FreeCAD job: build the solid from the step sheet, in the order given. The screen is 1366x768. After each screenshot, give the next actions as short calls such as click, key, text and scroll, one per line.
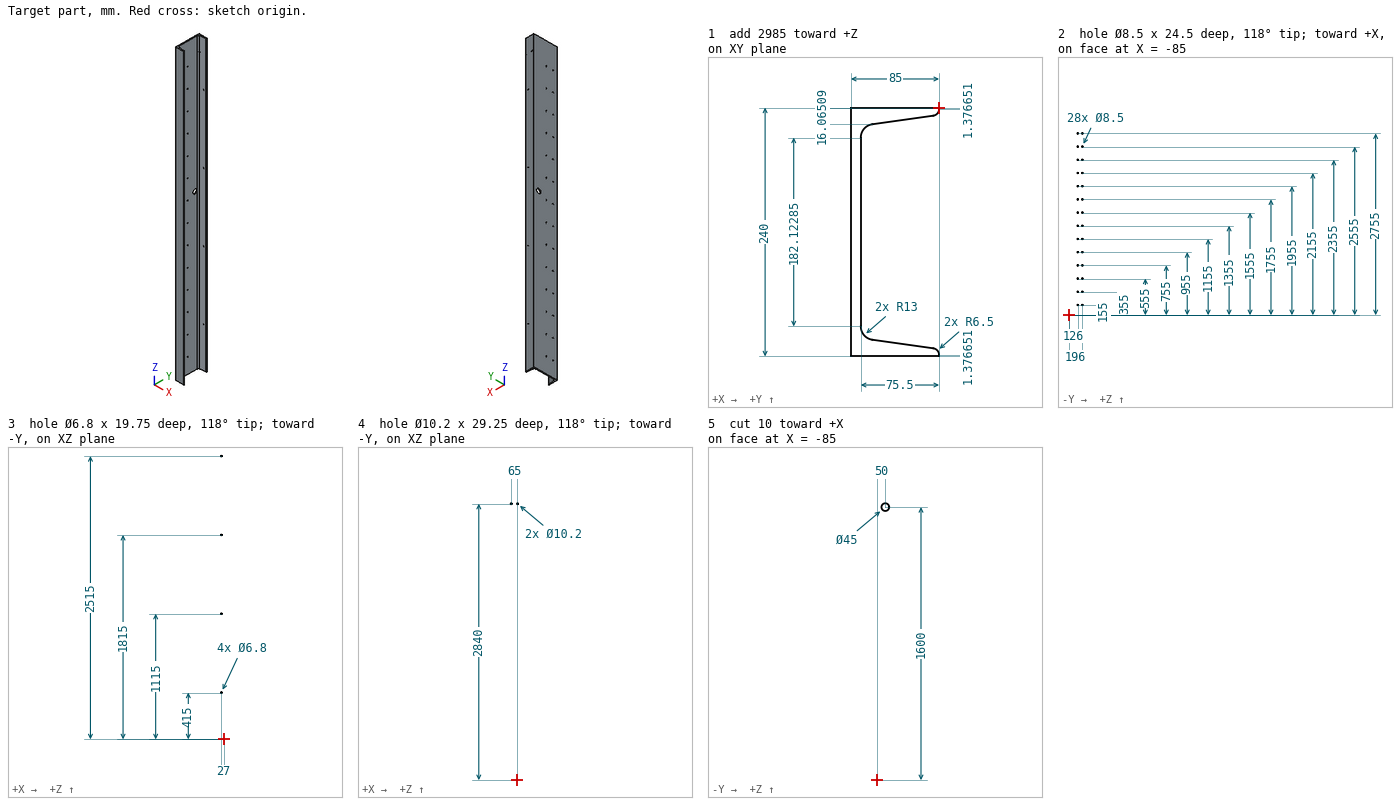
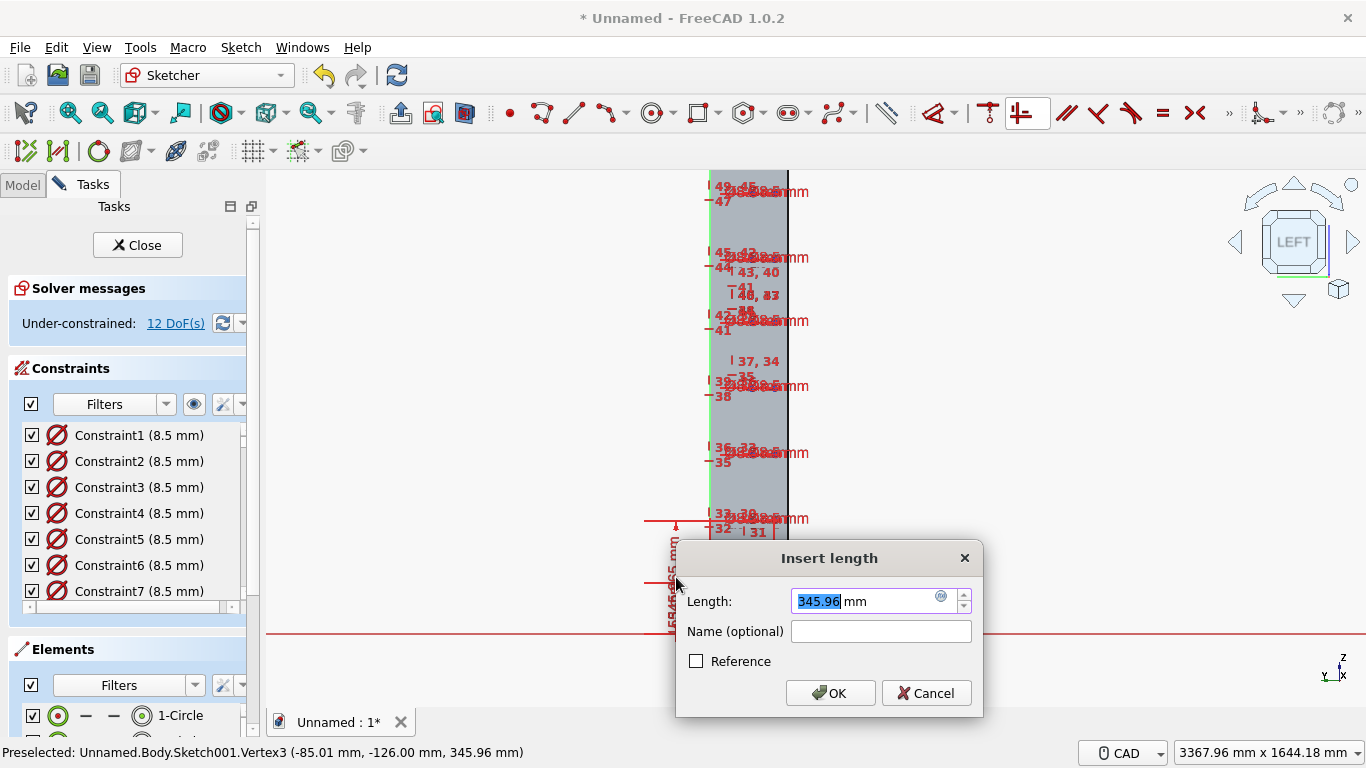
text(355)
key(Return)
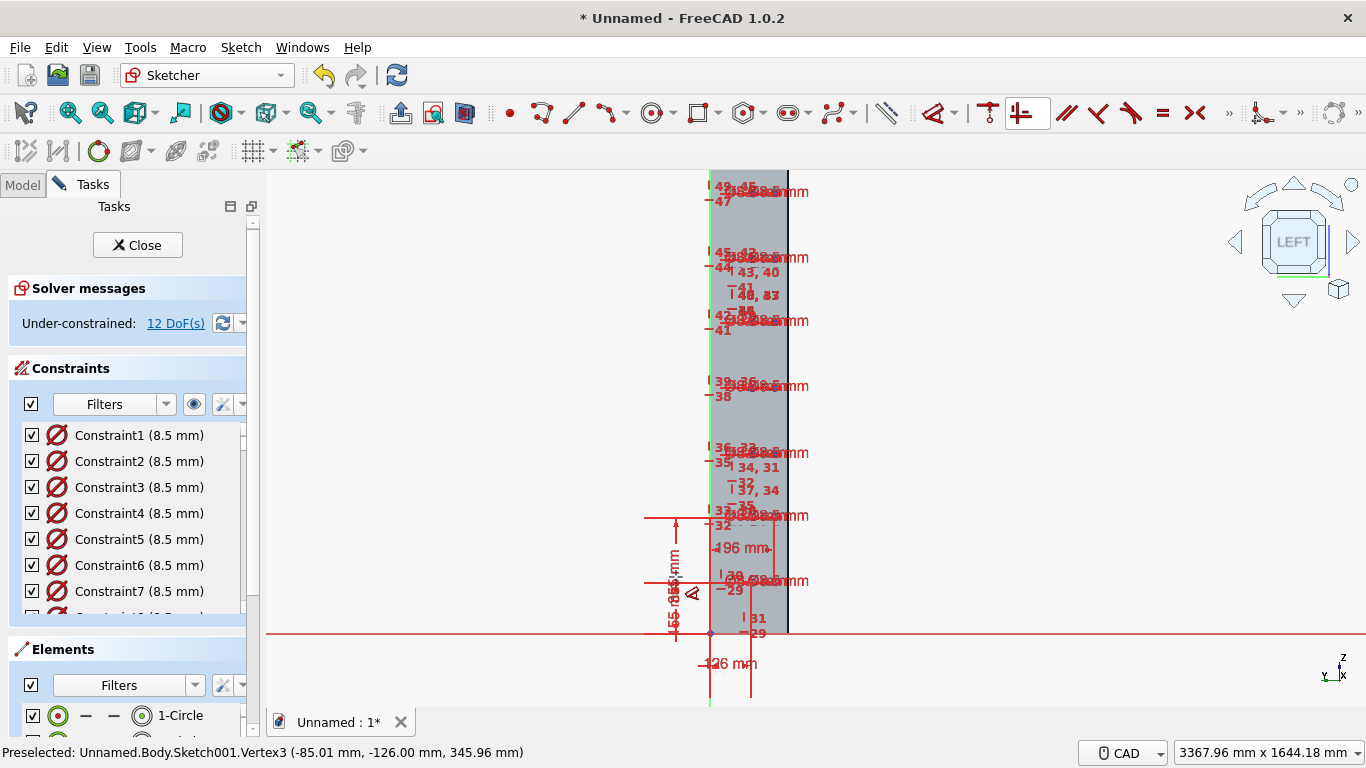
click(751, 455)
click(676, 503)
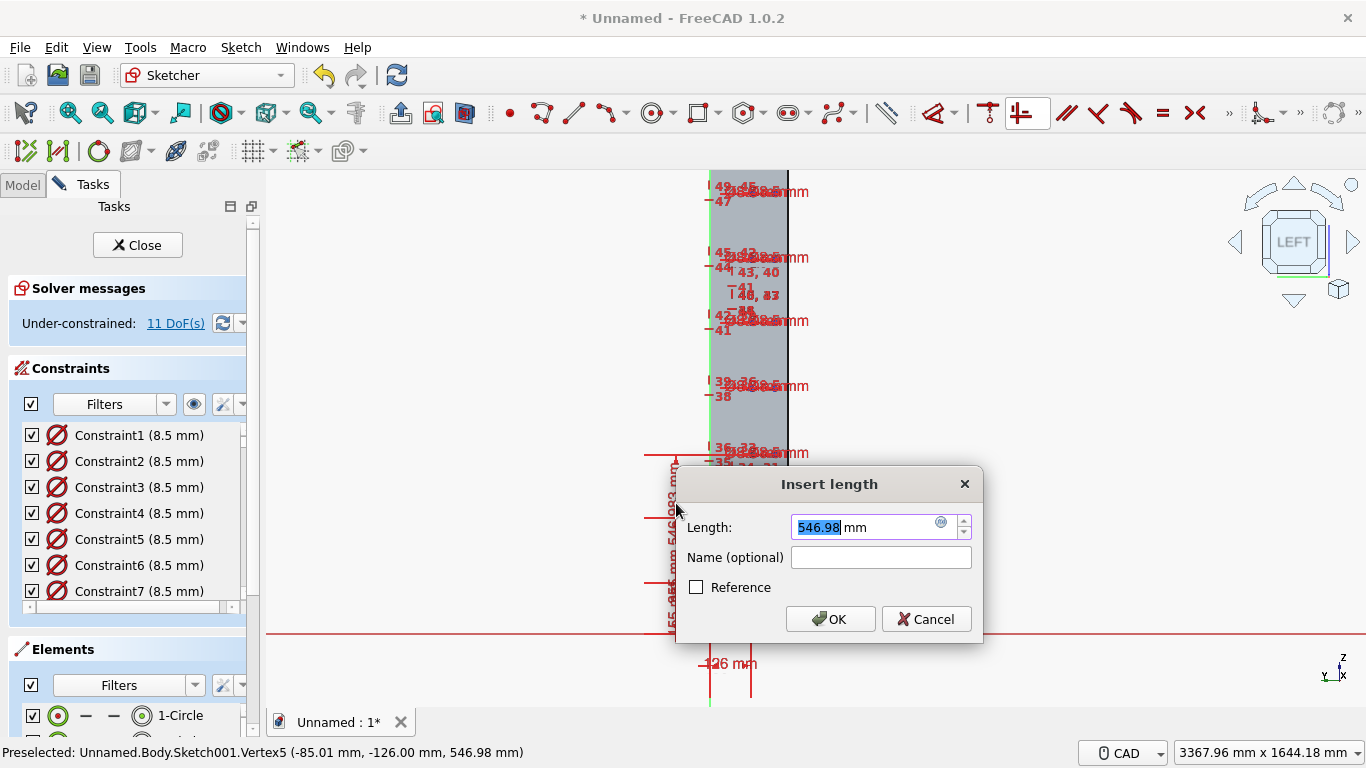
text(555)
key(Return)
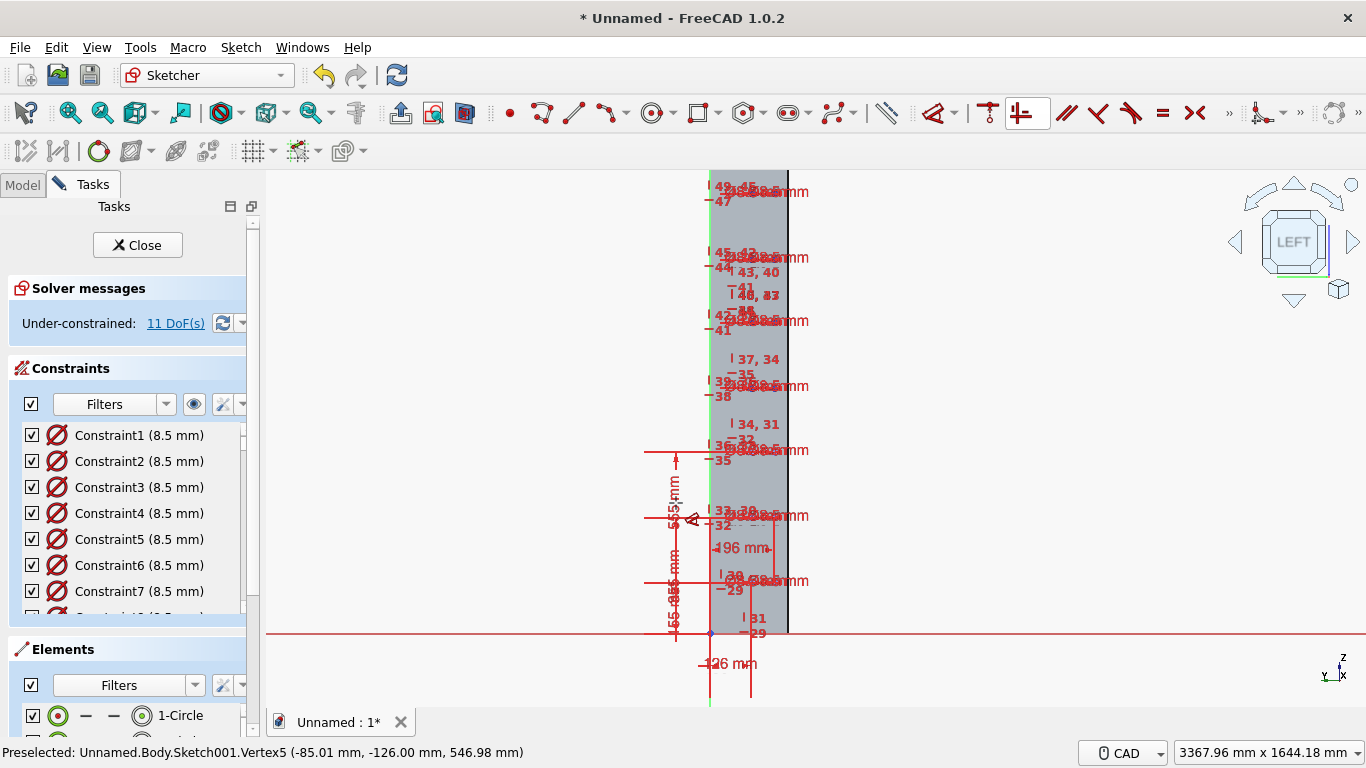
click(751, 388)
click(676, 454)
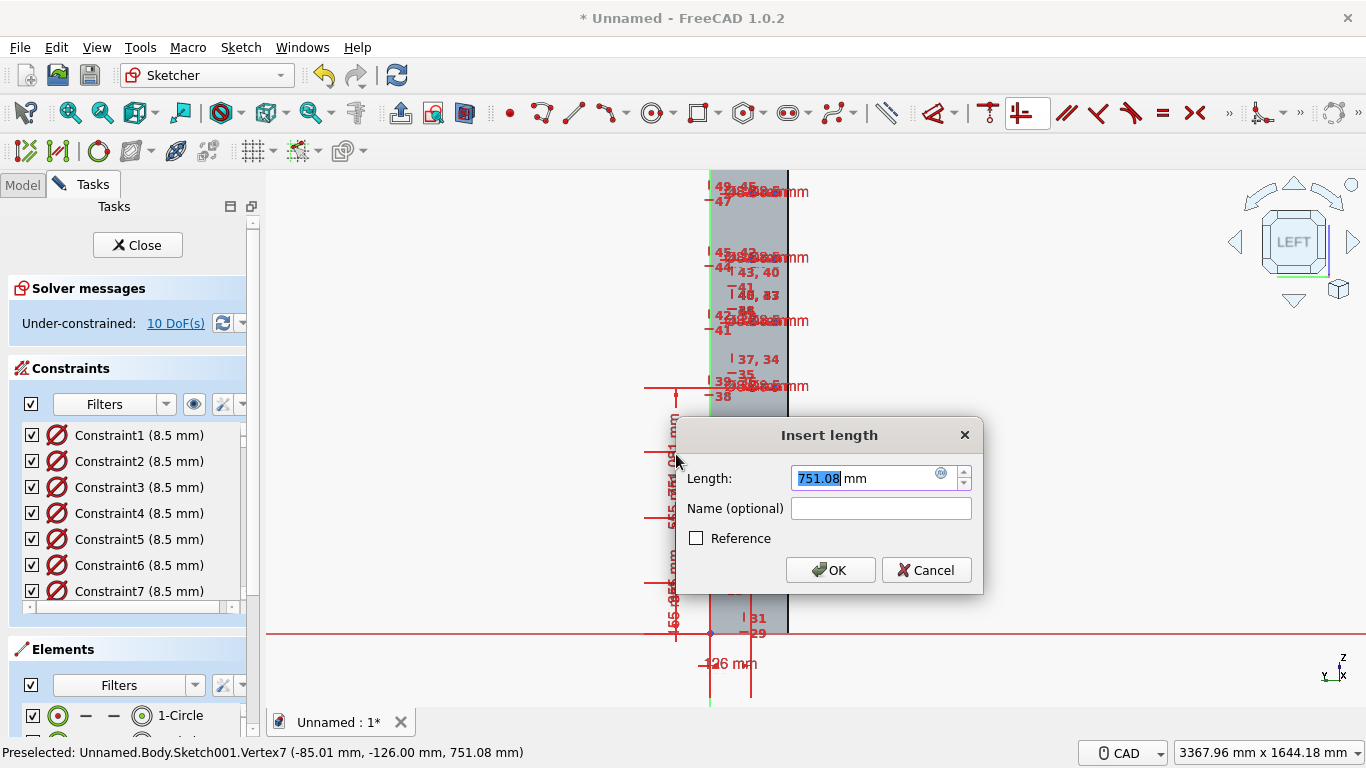
text(755)
key(Return)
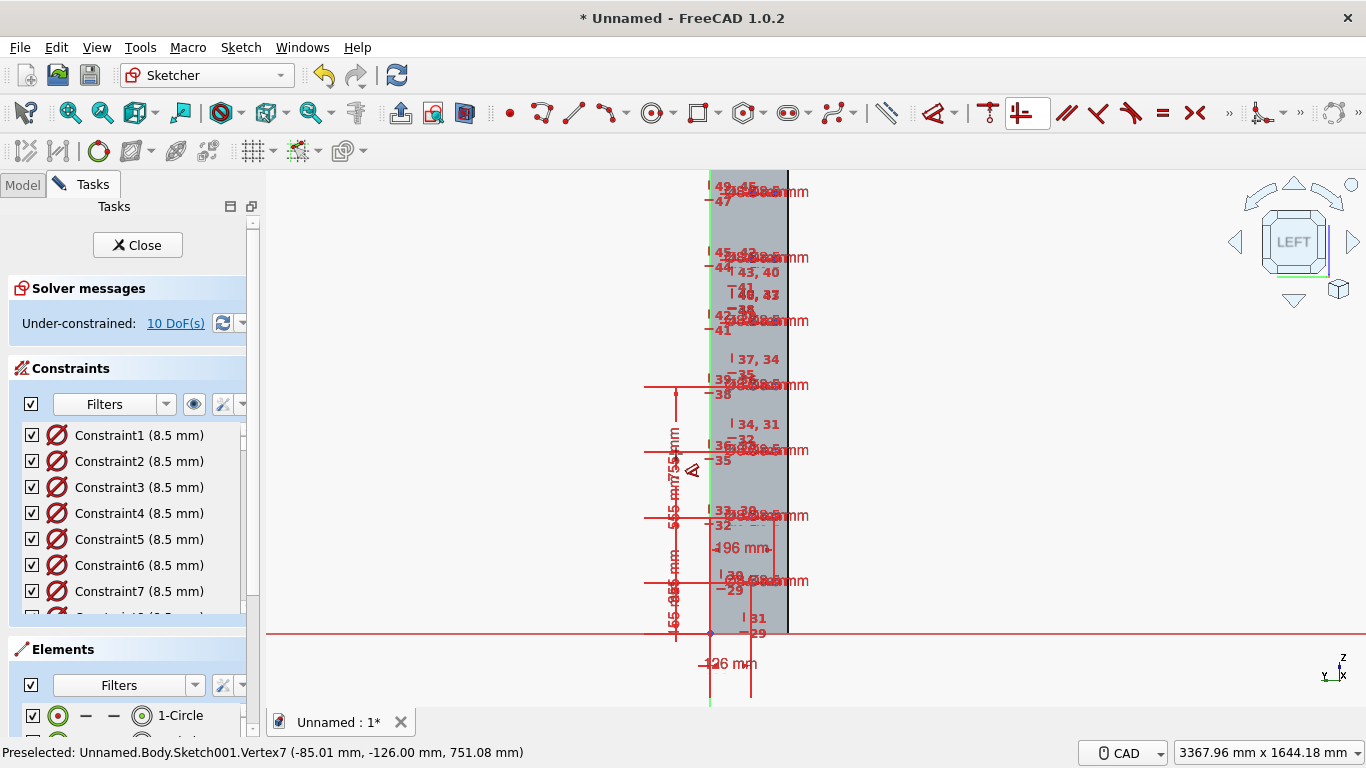
click(751, 323)
click(676, 478)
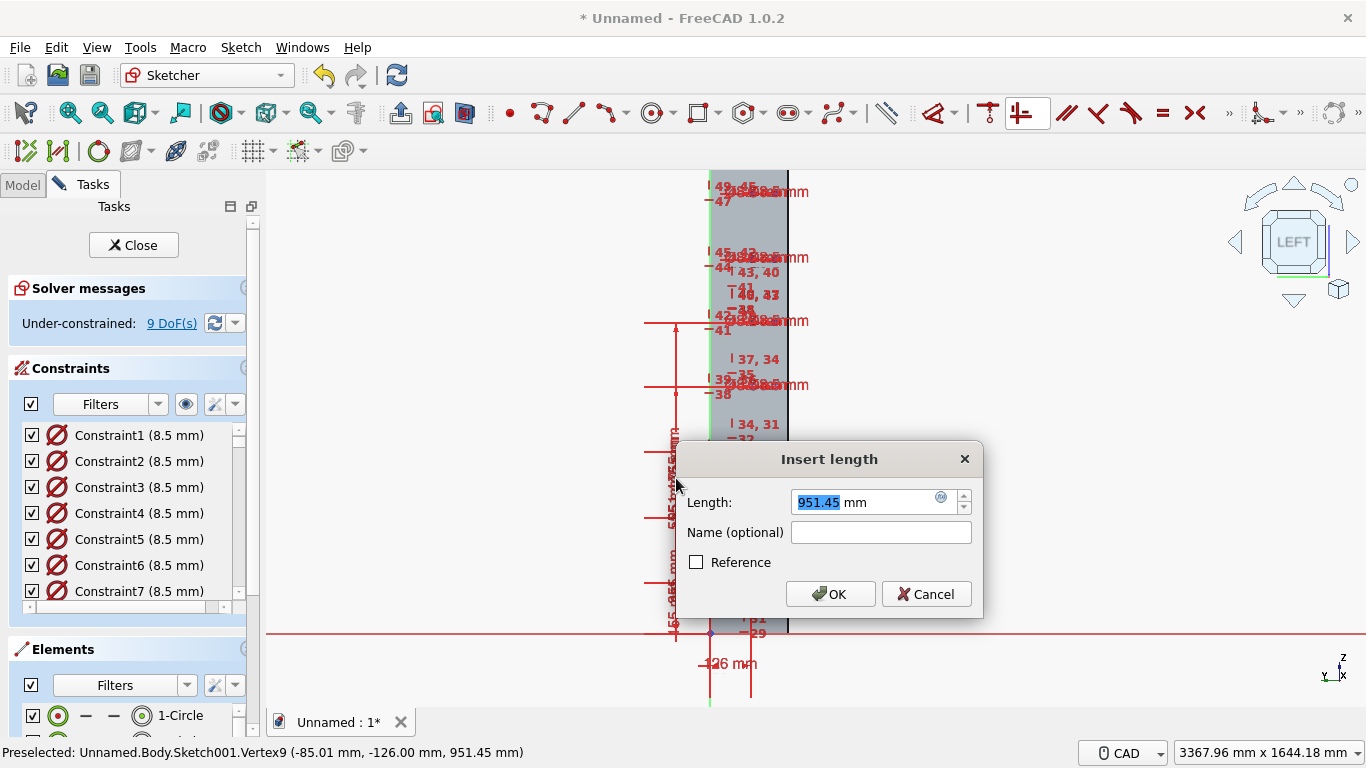
text(955)
key(Return)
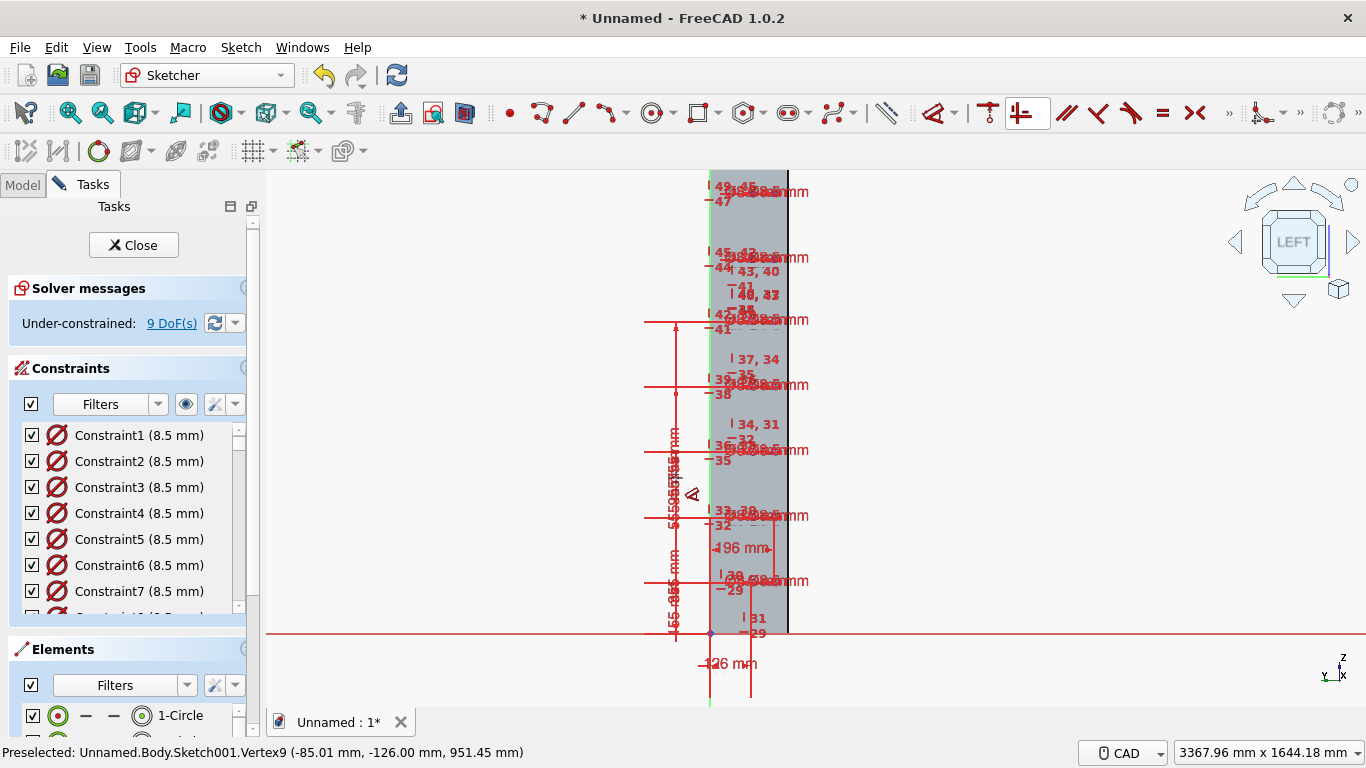
click(751, 260)
click(676, 360)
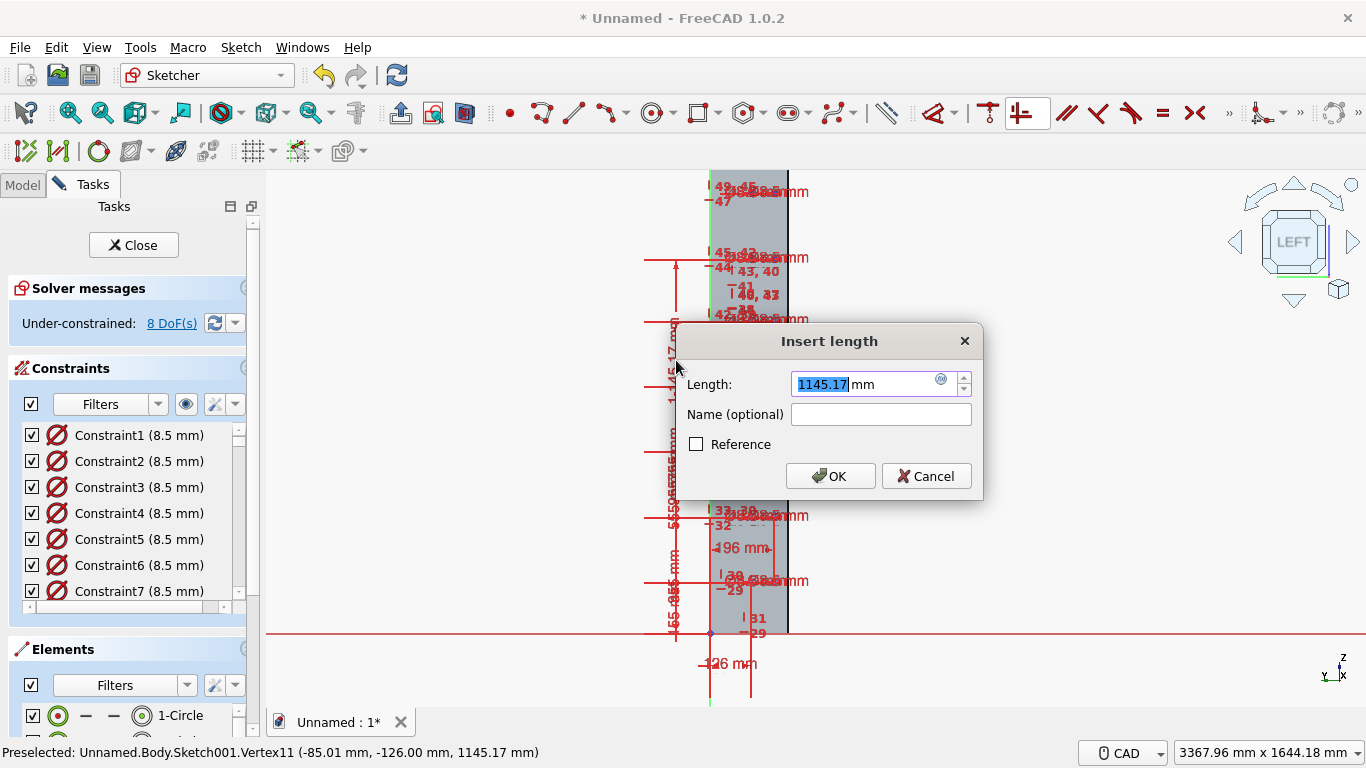
text(1155)
key(Return)